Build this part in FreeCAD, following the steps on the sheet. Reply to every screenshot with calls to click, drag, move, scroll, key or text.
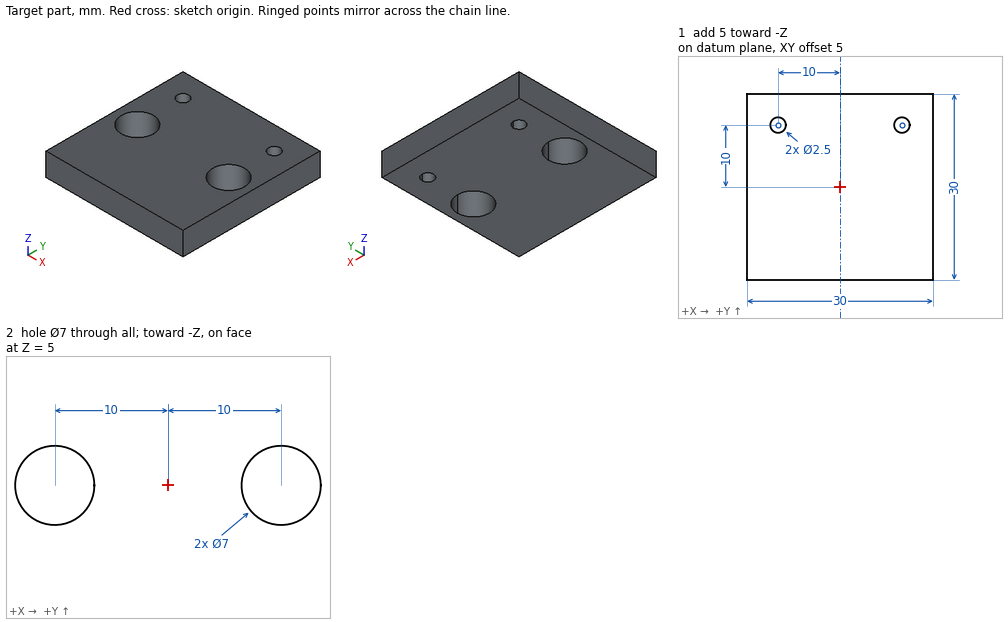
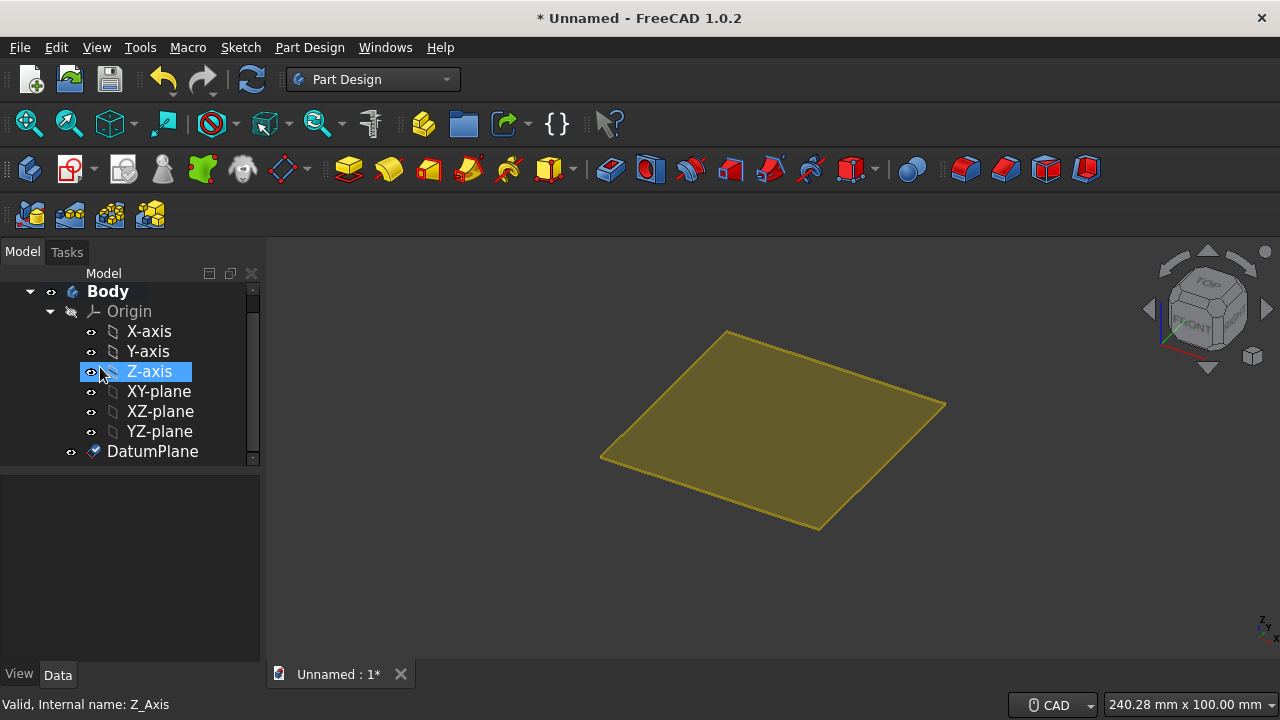
click(116, 452)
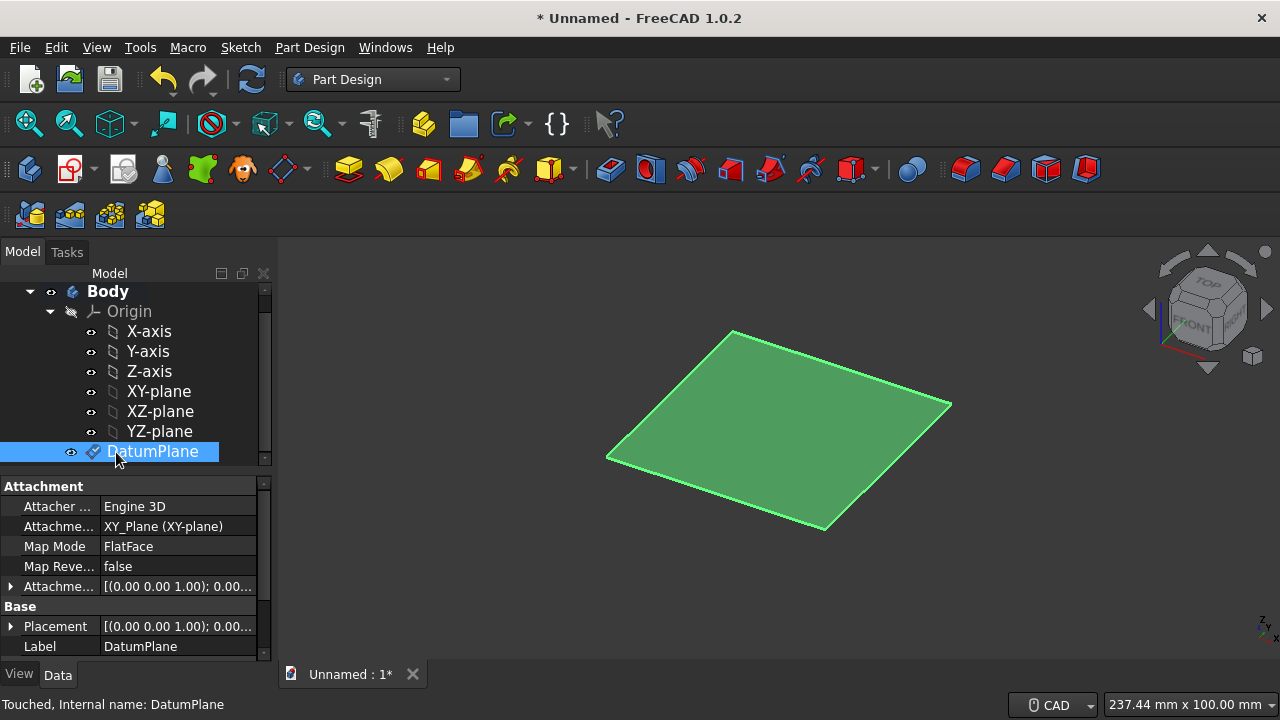
click(70, 170)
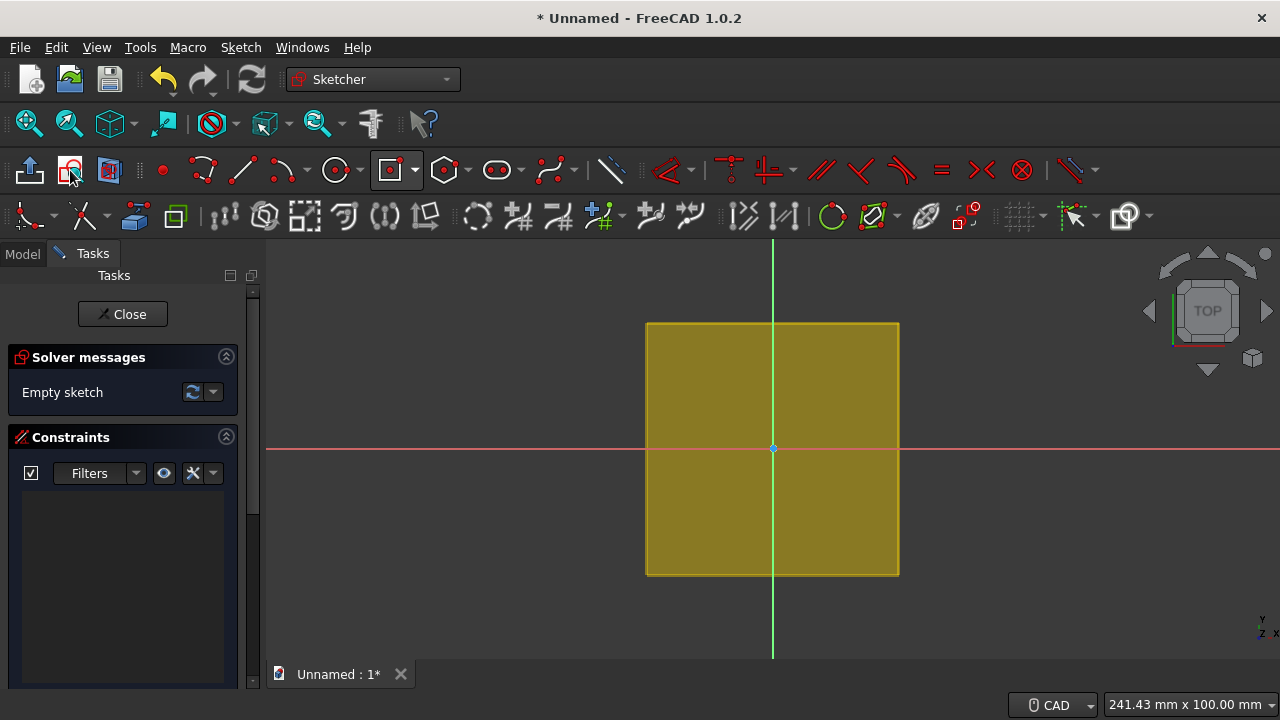
scroll(829, 449, up, 4)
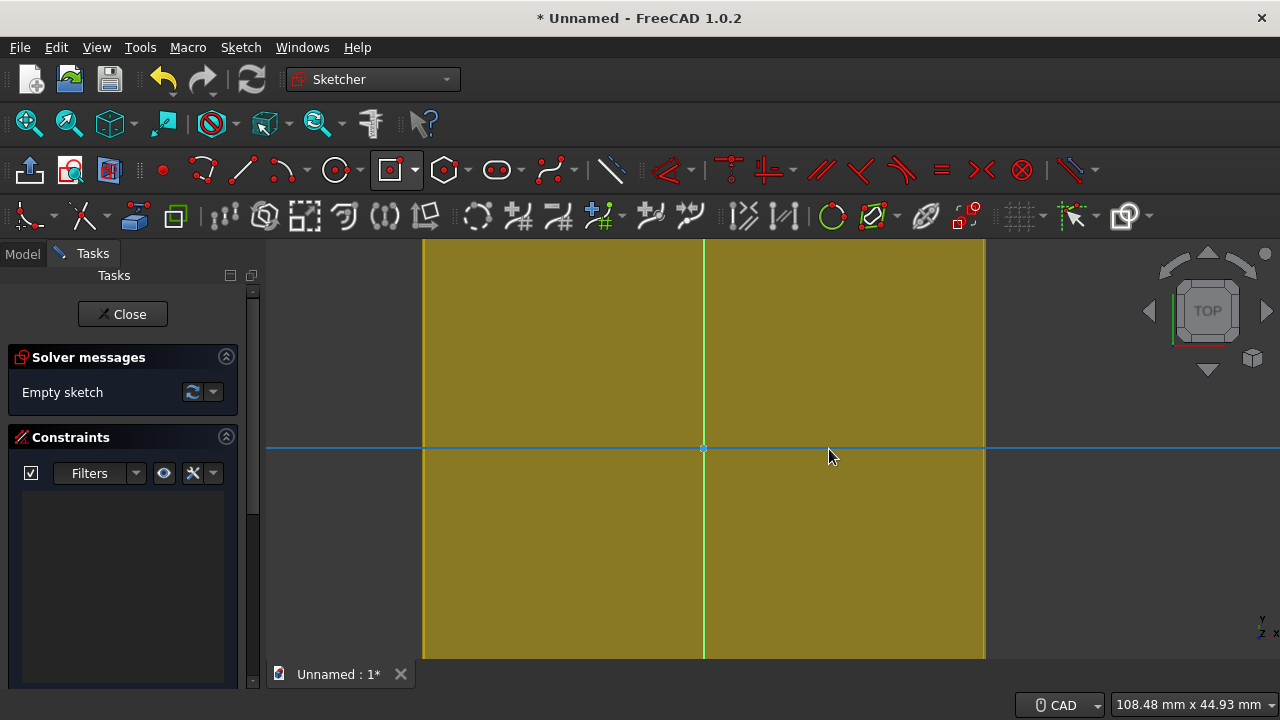
click(390, 170)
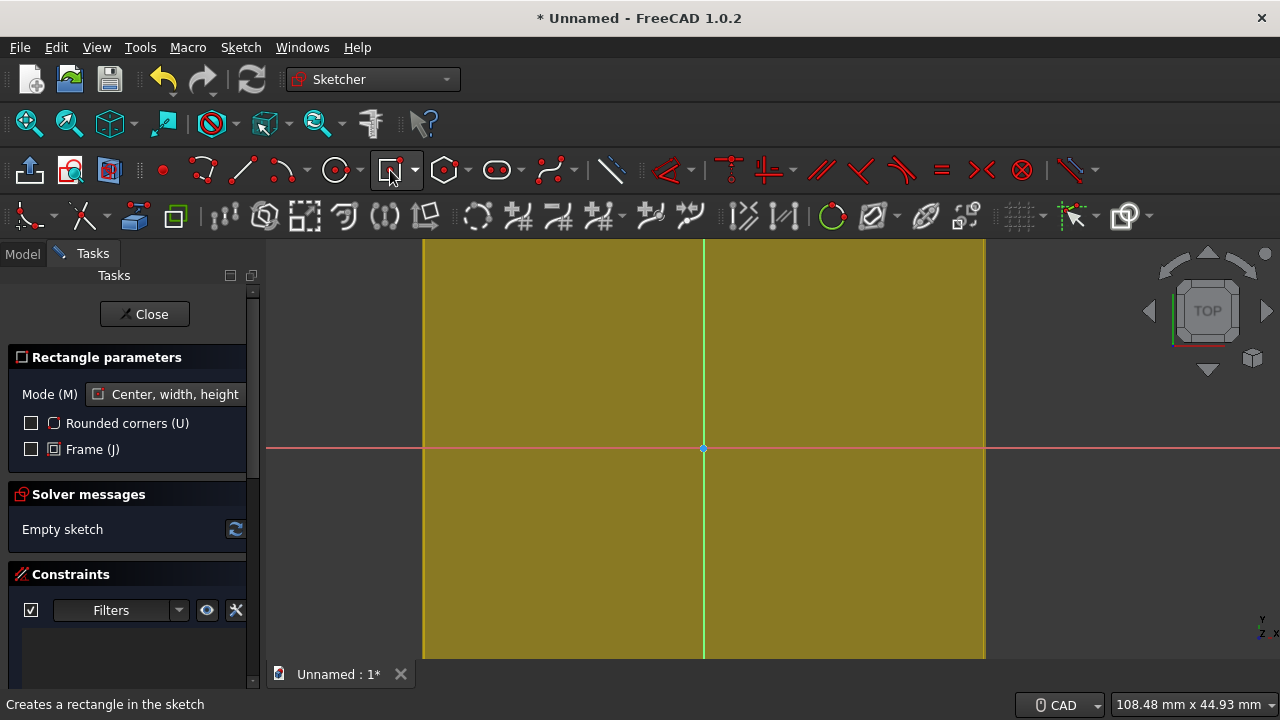
click(704, 448)
move(844, 308)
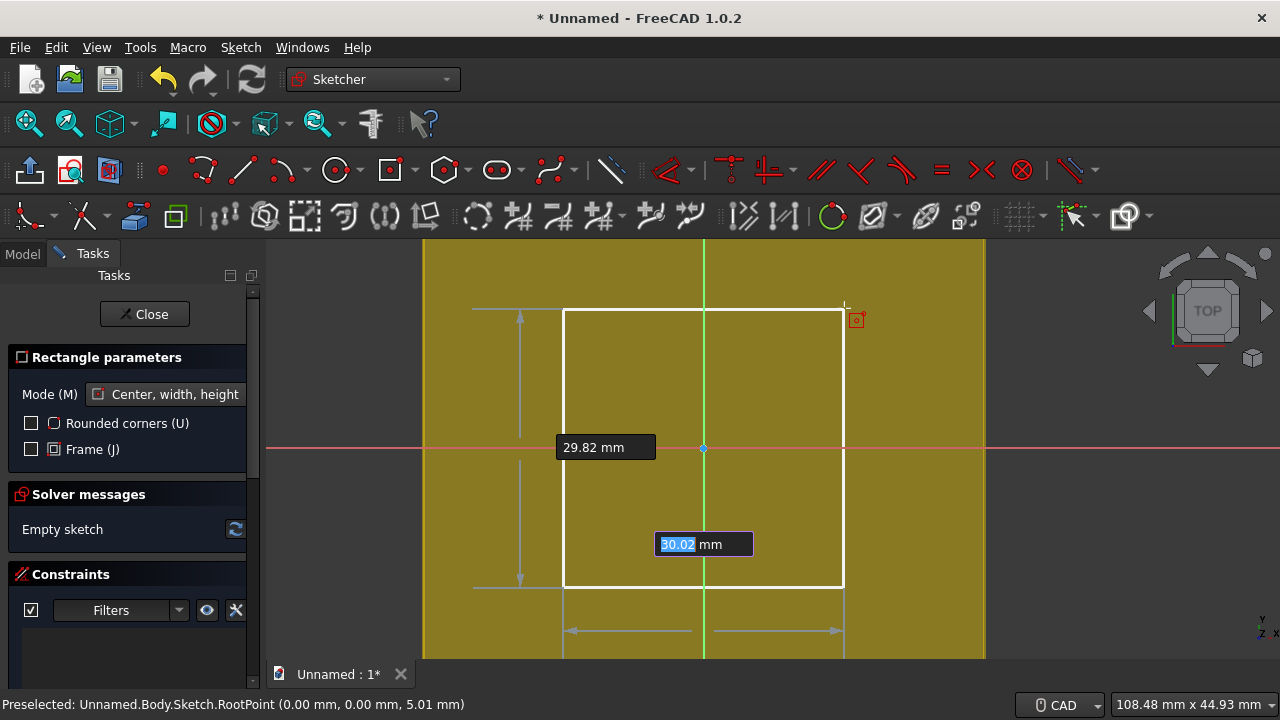
text(30)
key(Tab)
text(30)
key(Return)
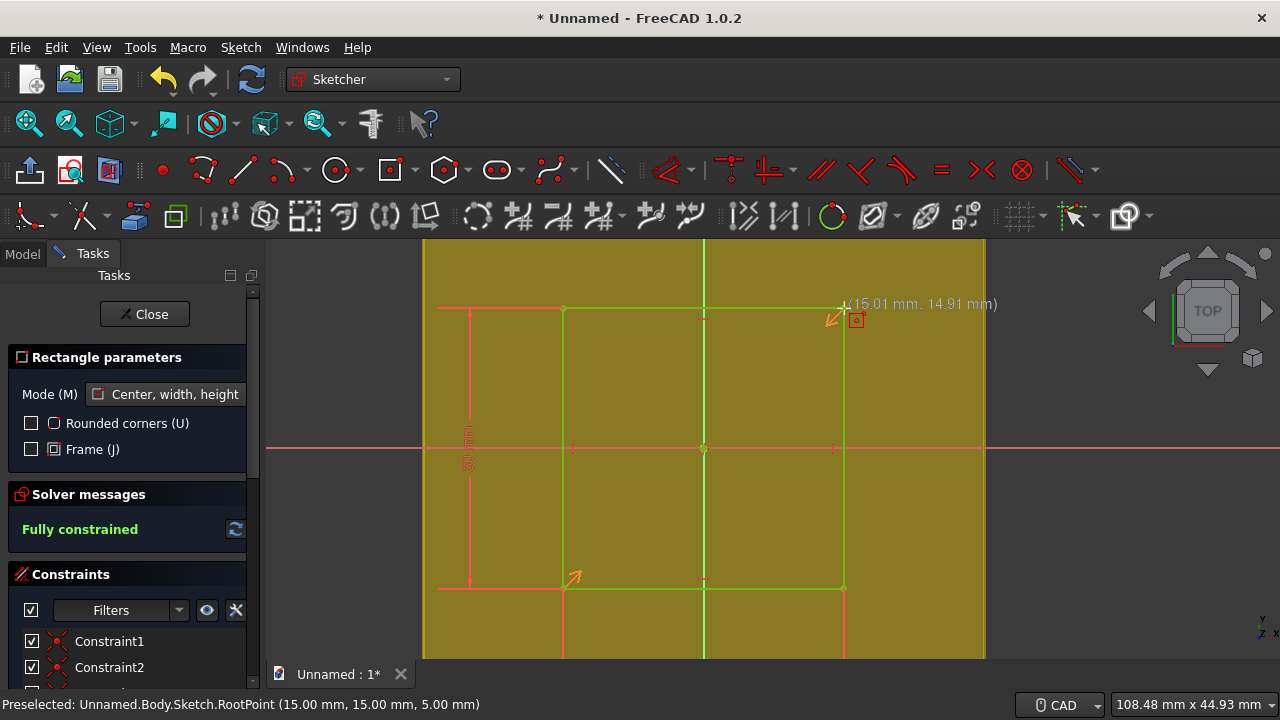
key(g)
key(c)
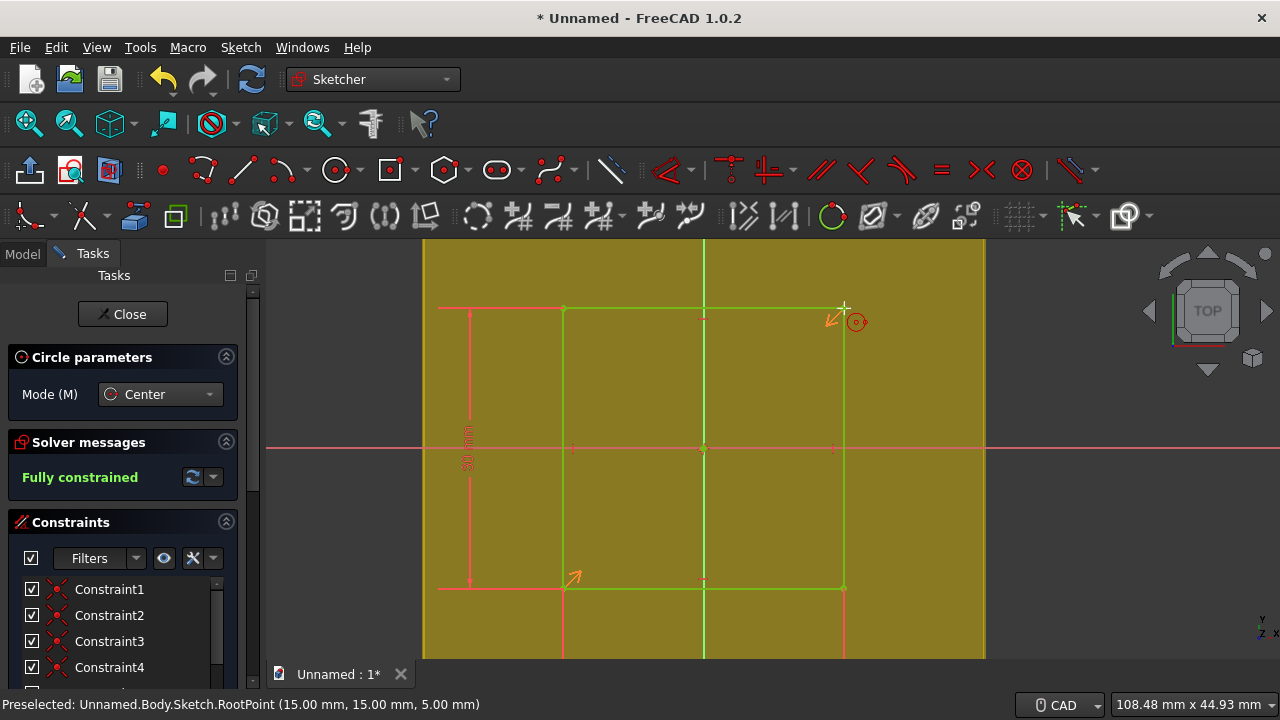
scroll(610, 355, up, 4)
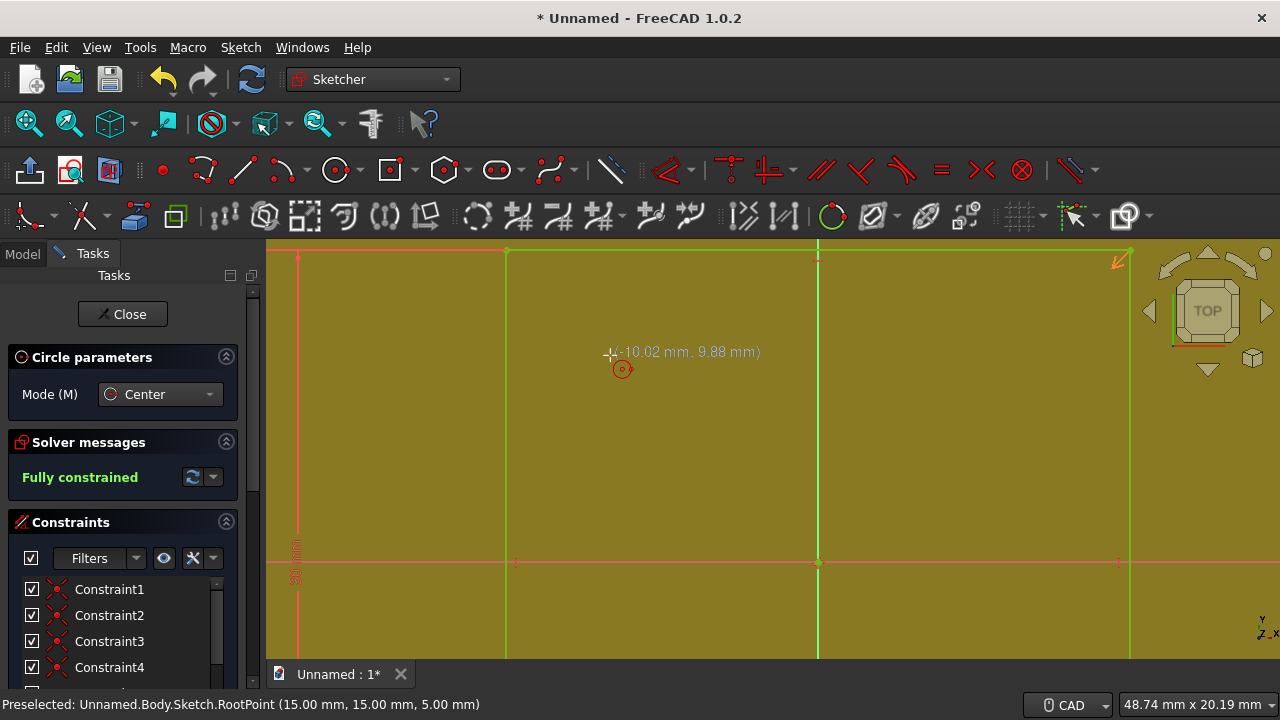
click(610, 354)
move(628, 336)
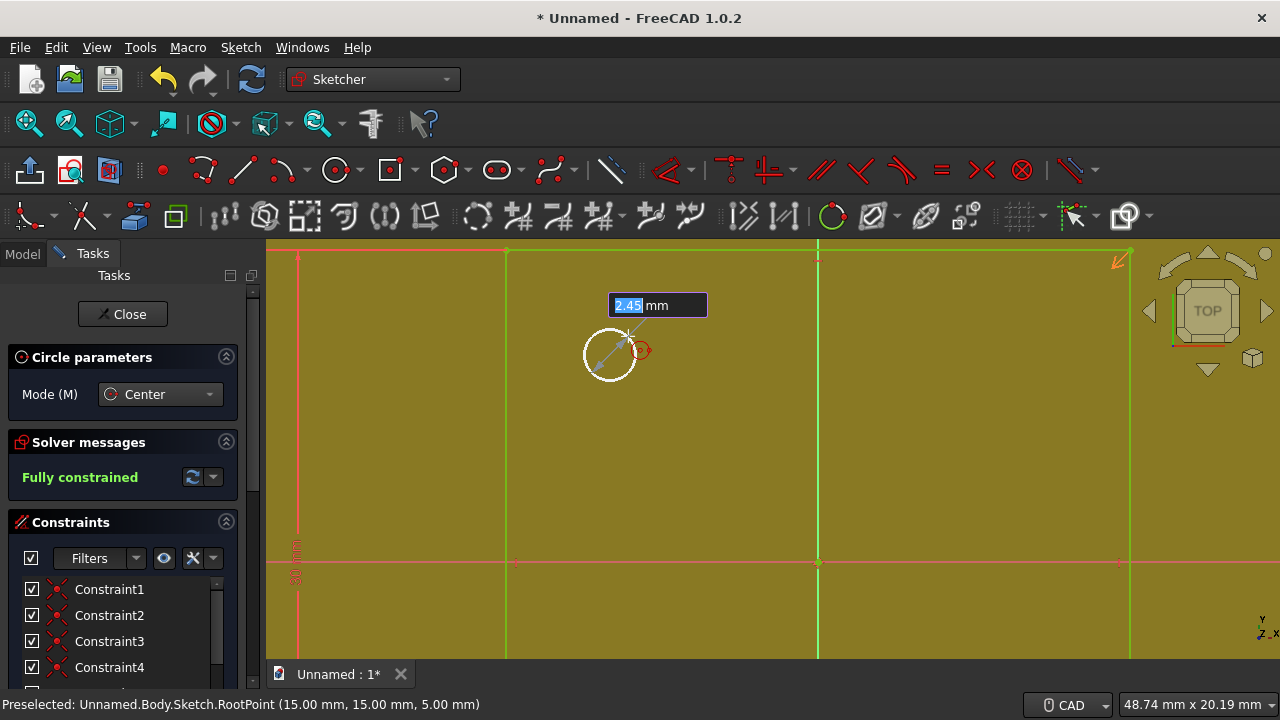
text(2.5)
key(Return)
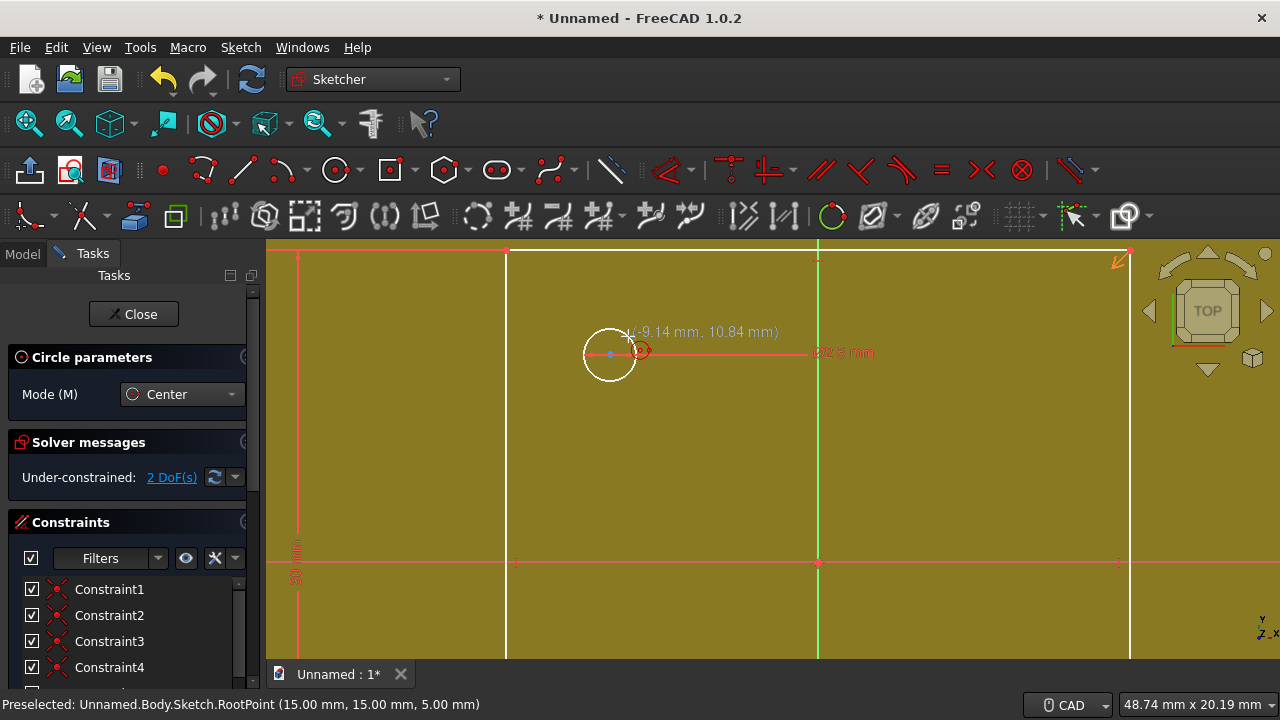
click(1026, 354)
move(1045, 336)